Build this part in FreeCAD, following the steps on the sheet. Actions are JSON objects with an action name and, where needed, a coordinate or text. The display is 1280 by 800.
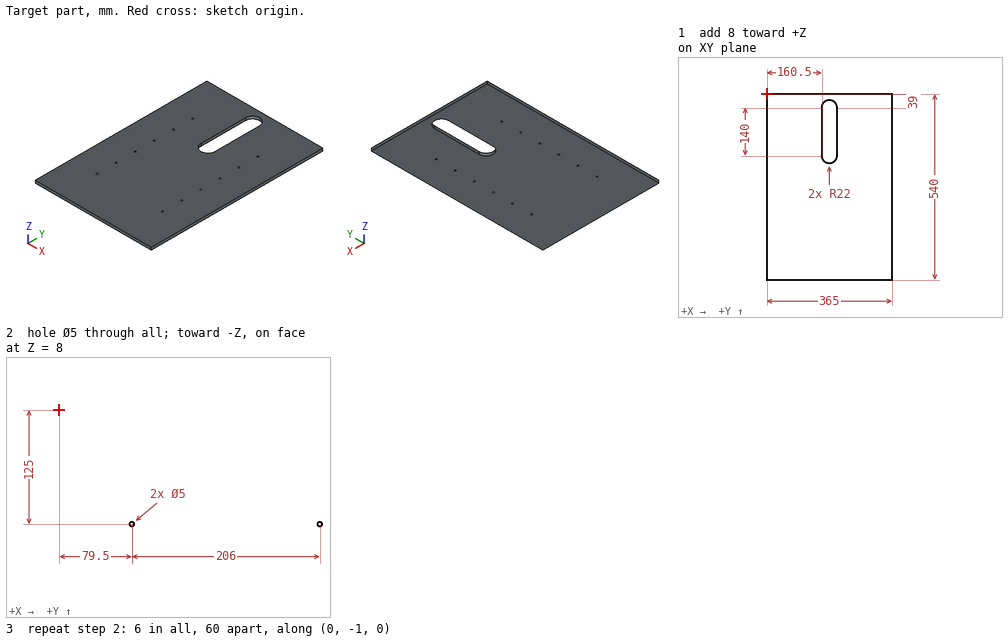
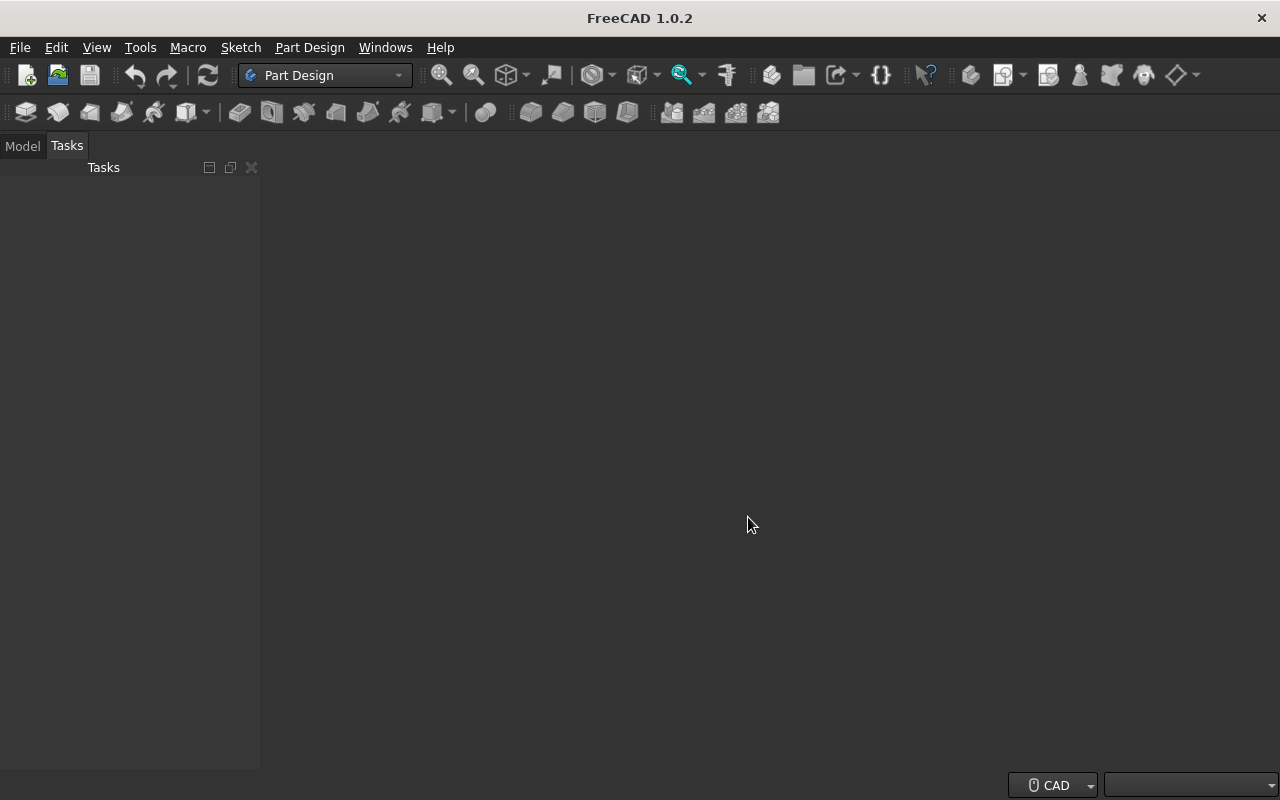
{"action": "left_click", "coordinate": [26, 76]}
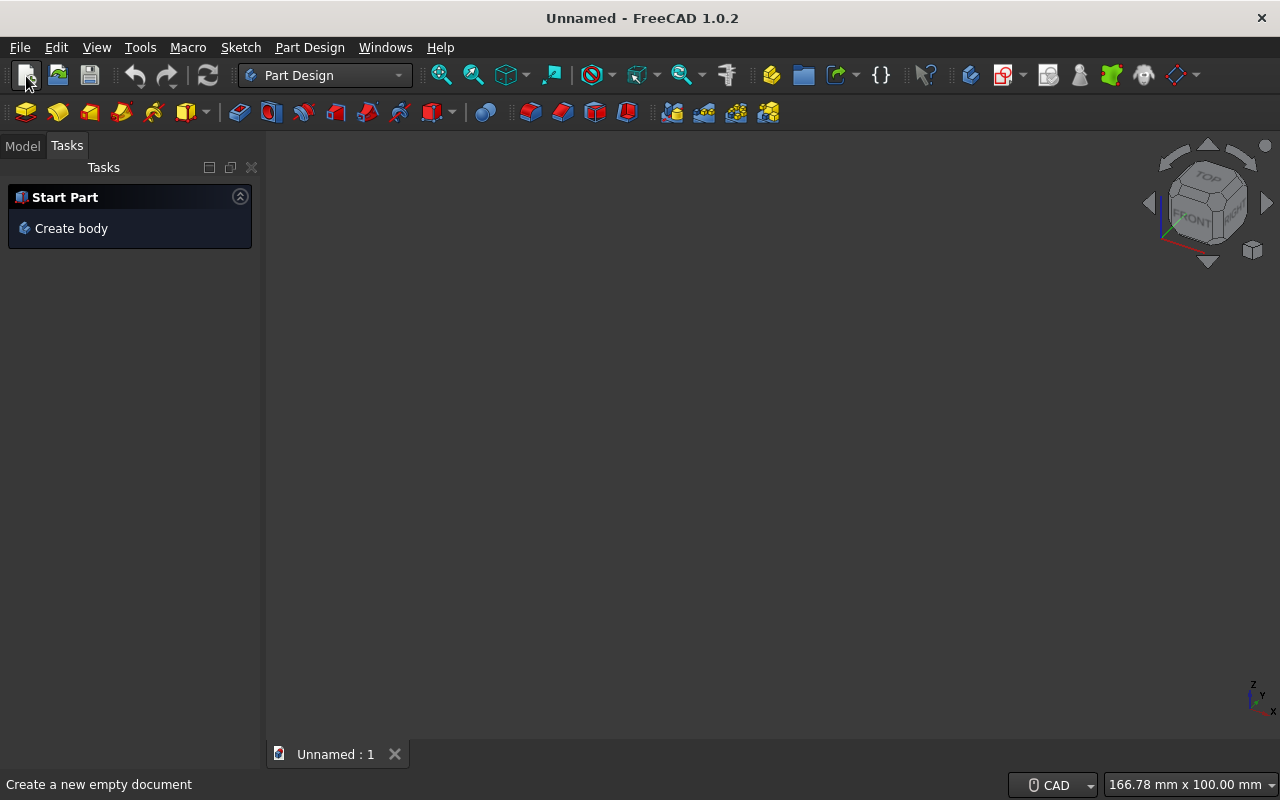
{"action": "left_click", "coordinate": [1004, 76]}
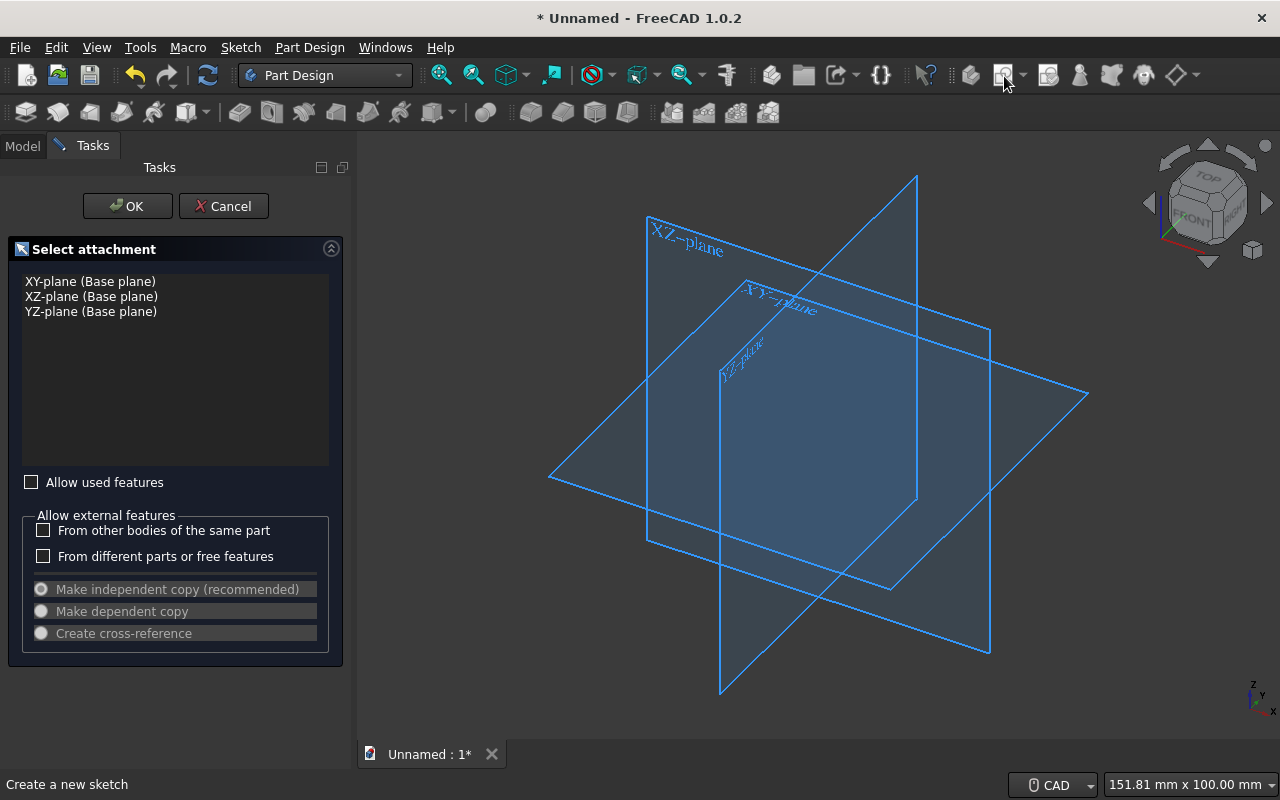
{"action": "left_click", "coordinate": [82, 282]}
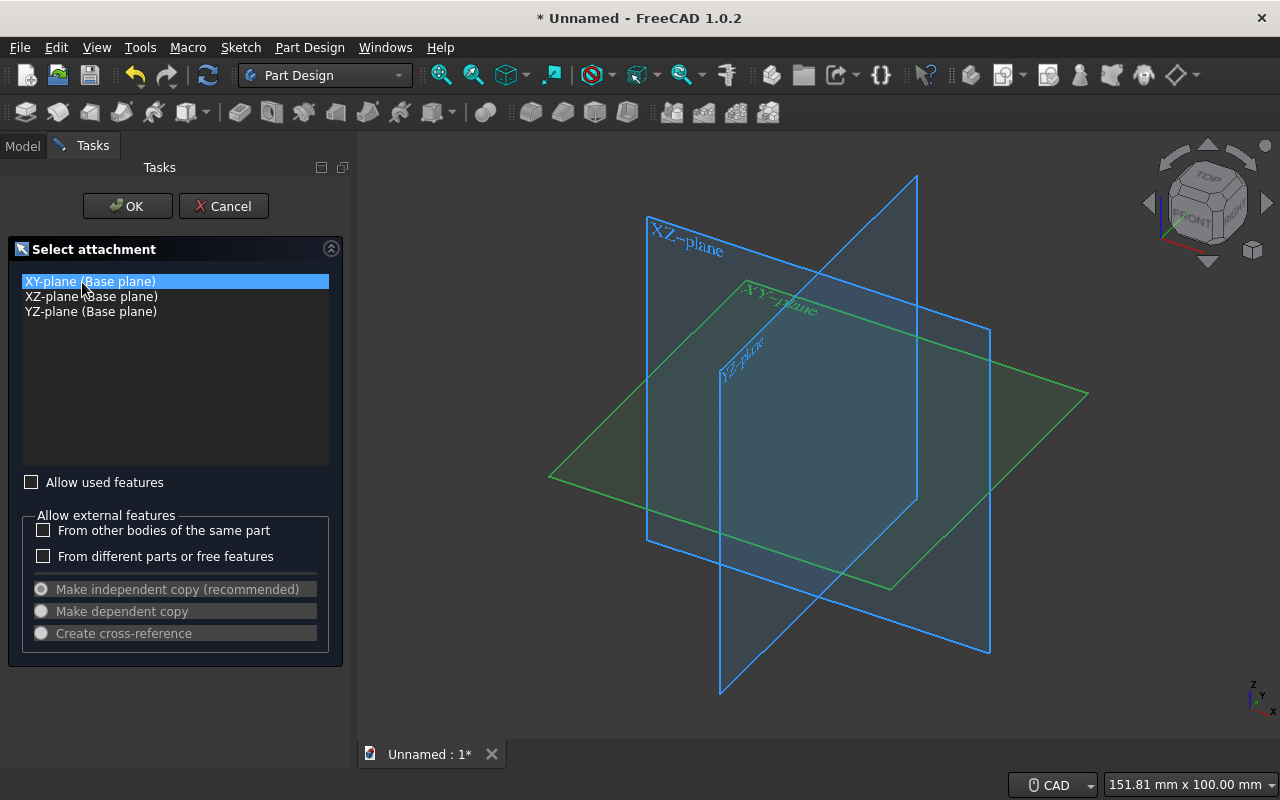
{"action": "left_click", "coordinate": [128, 206]}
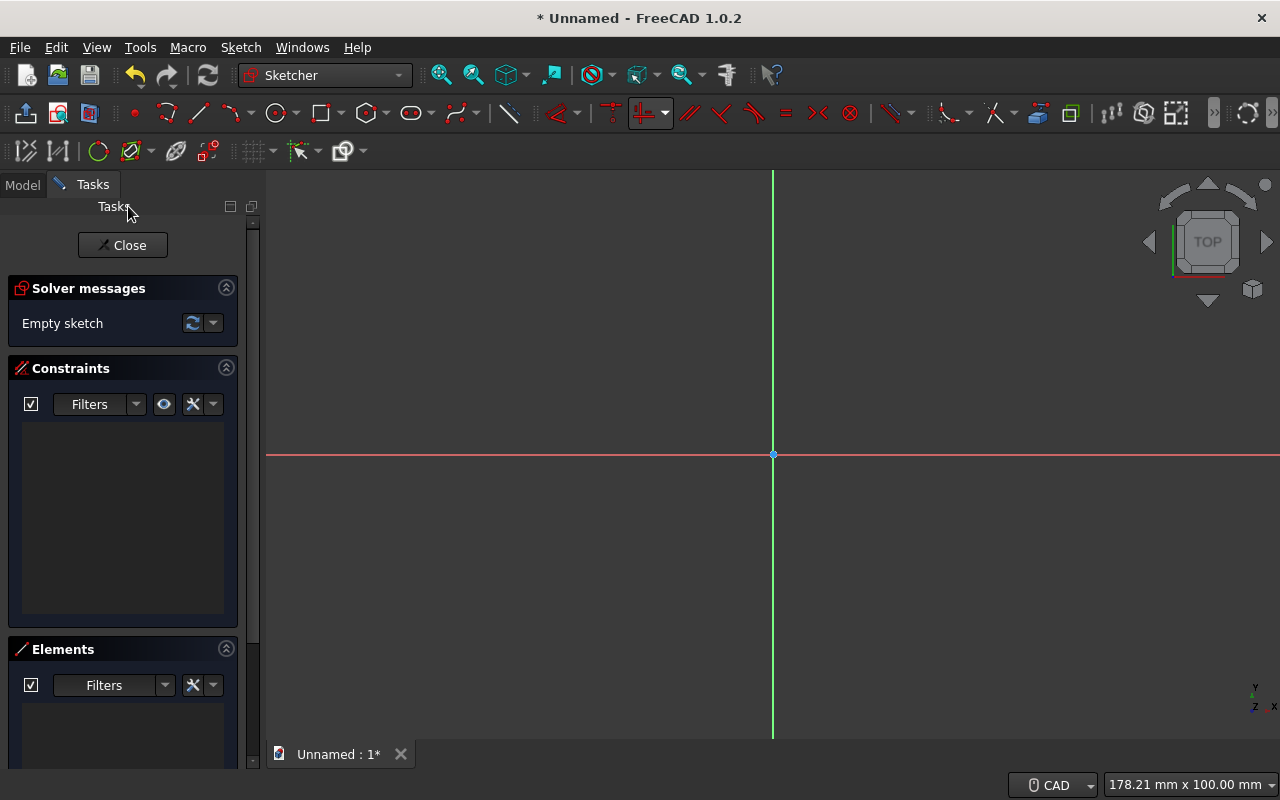
{"action": "scroll", "coordinate": [567, 263], "scroll_direction": "down", "scroll_amount": 11}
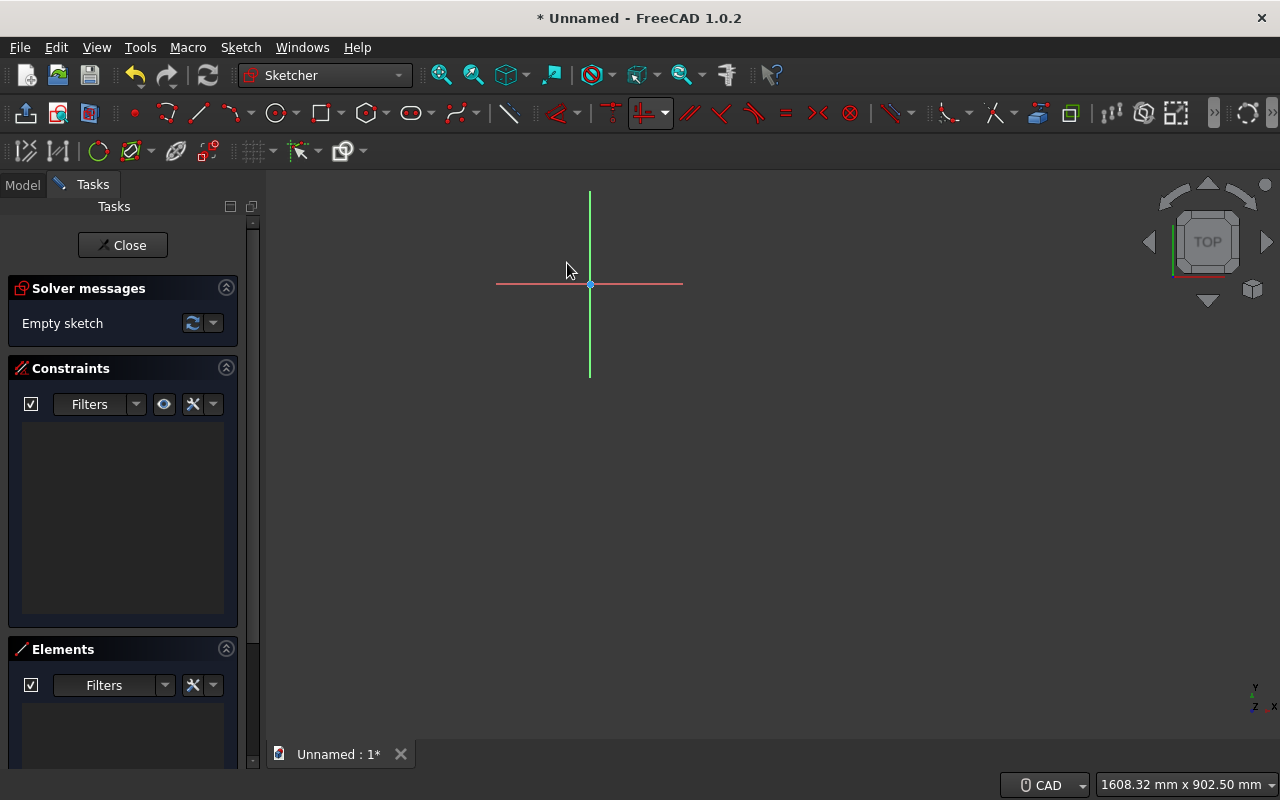
{"action": "left_click", "coordinate": [322, 114]}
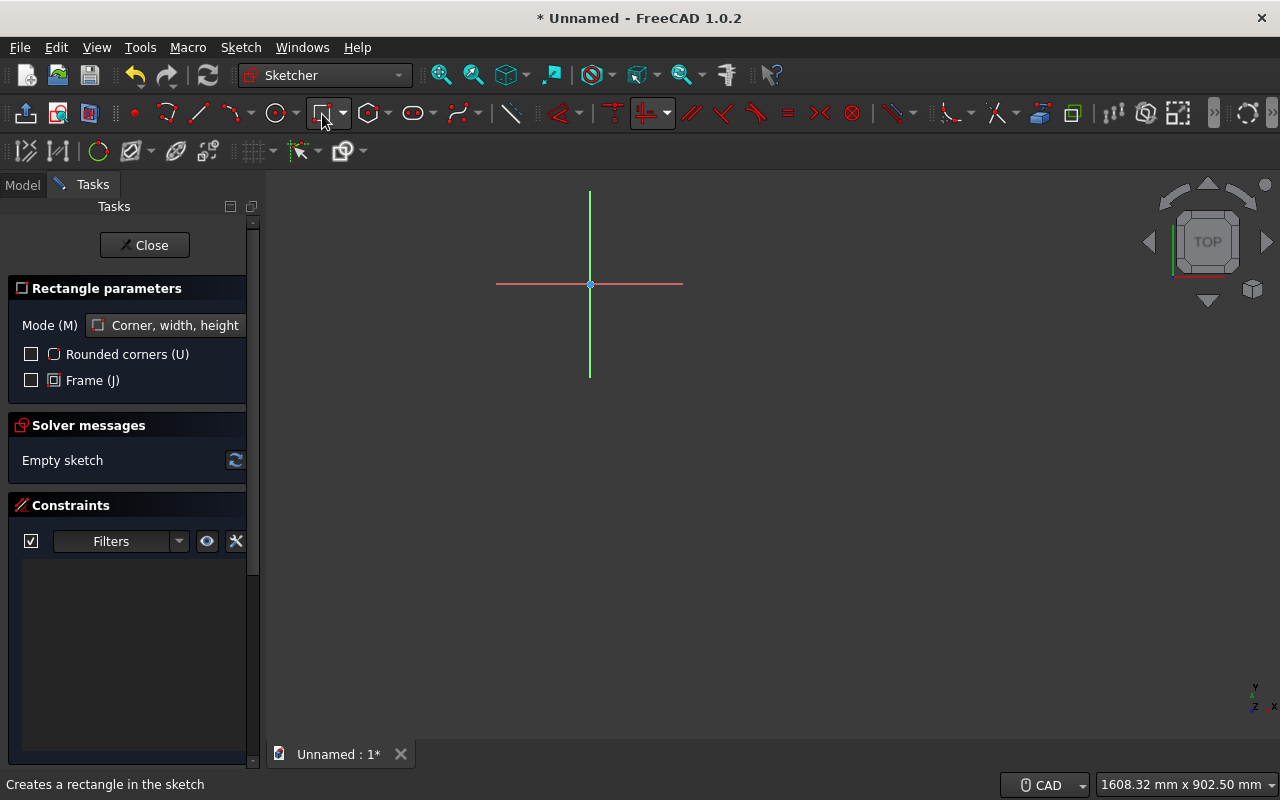
{"action": "left_click", "coordinate": [590, 284]}
{"action": "mouse_move", "coordinate": [820, 625]}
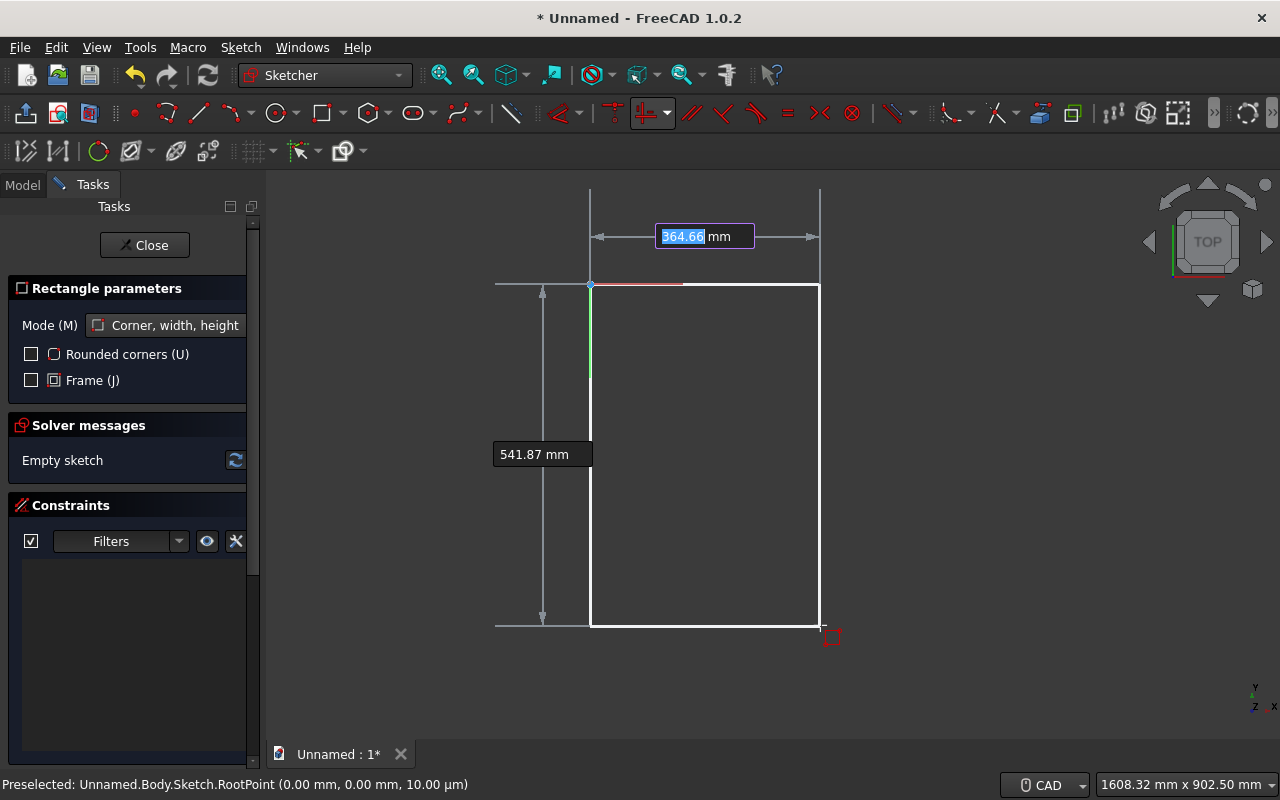
{"action": "type", "text": "365"}
{"action": "key", "text": "Tab"}
{"action": "type", "text": "540"}
{"action": "key", "text": "Return"}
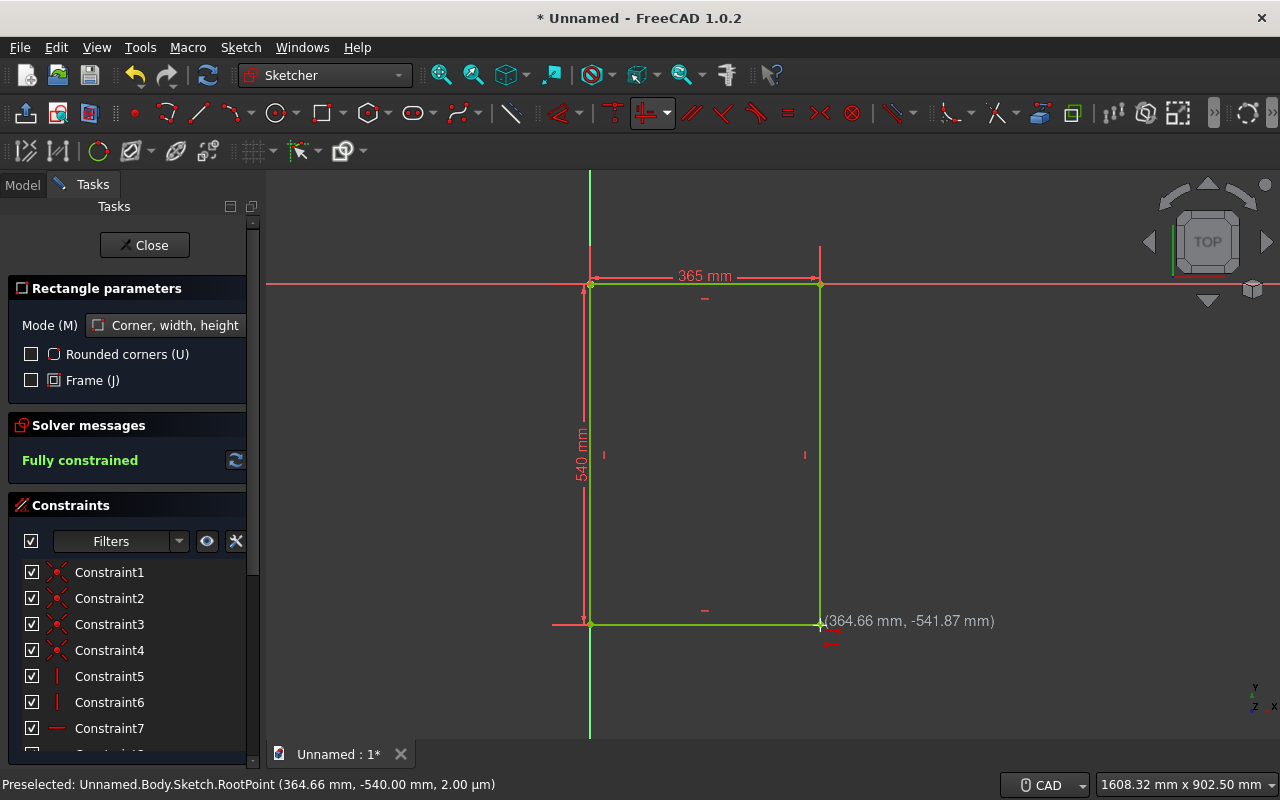
{"action": "left_click", "coordinate": [414, 114]}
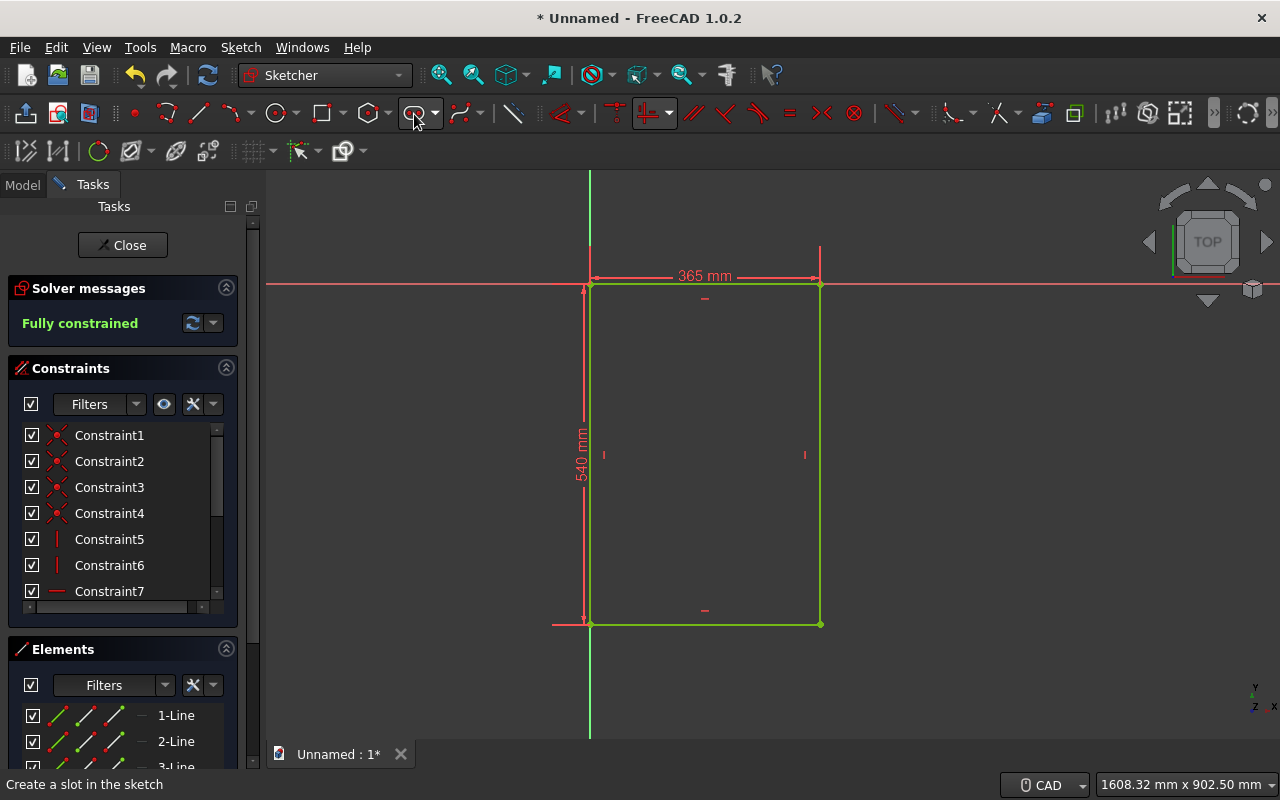
{"action": "scroll", "coordinate": [705, 397], "scroll_direction": "up", "scroll_amount": 3}